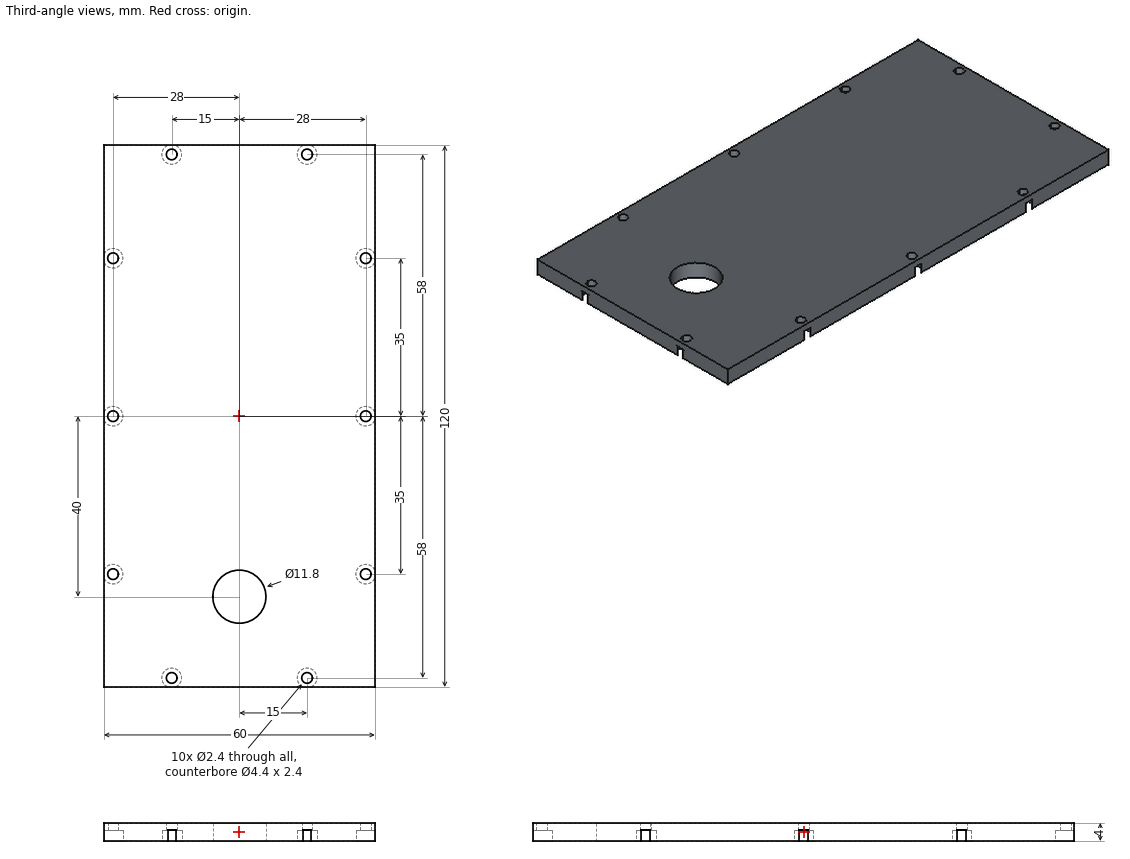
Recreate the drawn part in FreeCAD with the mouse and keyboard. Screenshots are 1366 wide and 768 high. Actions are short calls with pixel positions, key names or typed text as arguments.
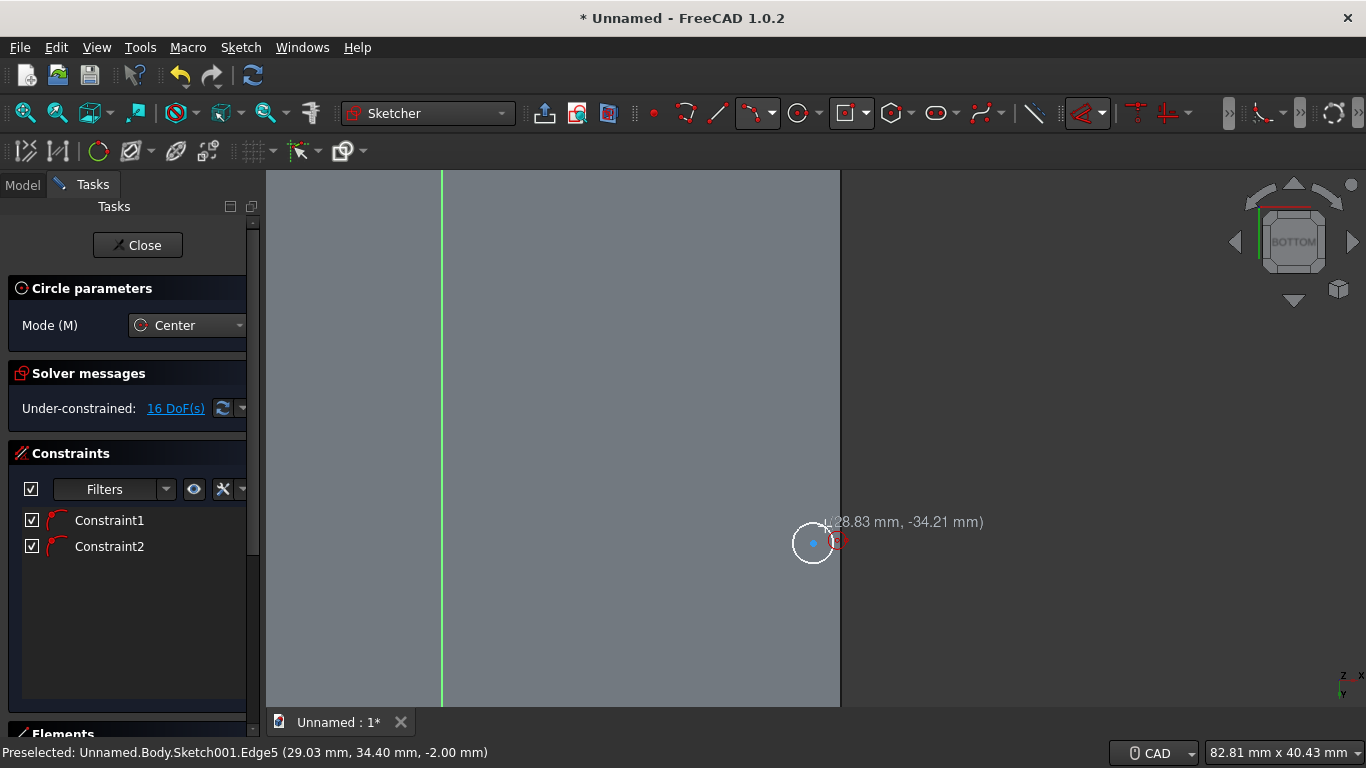
scroll(825, 531, down, 8)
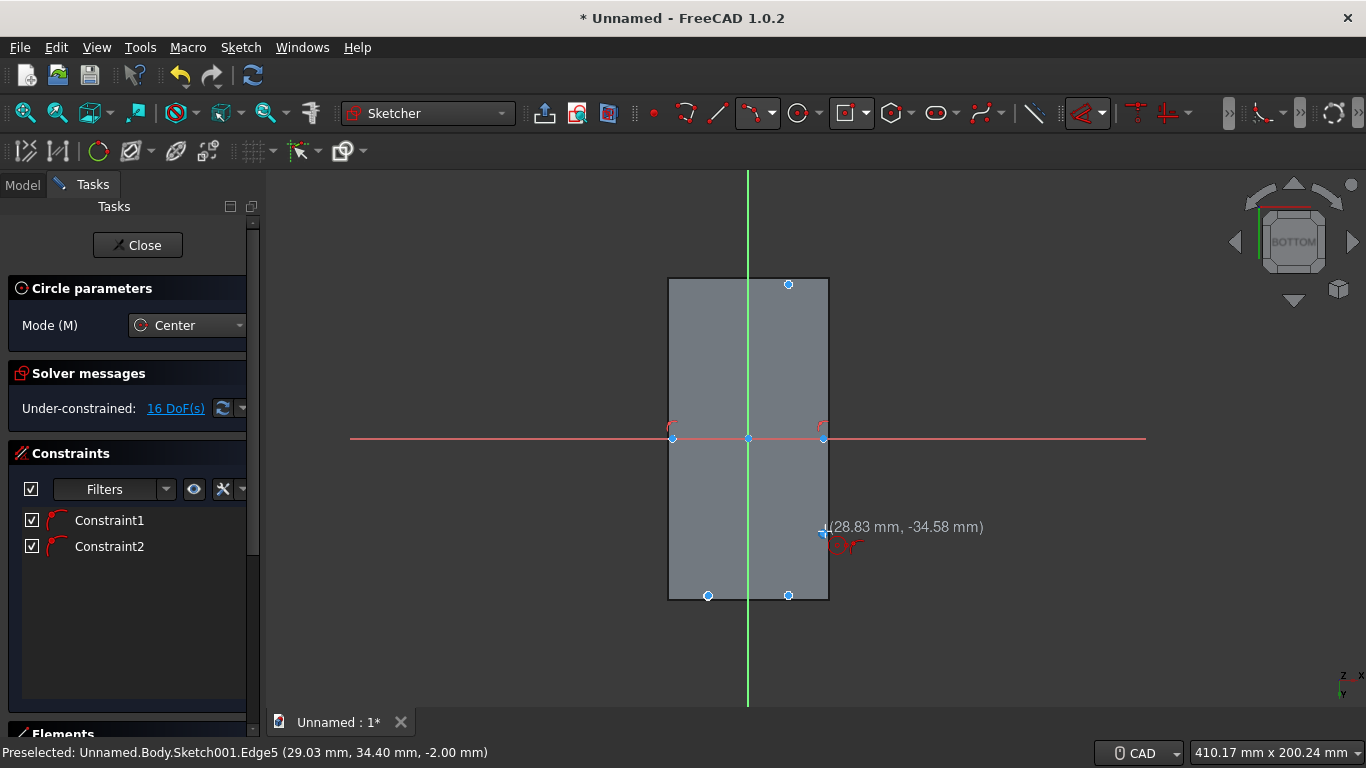
scroll(673, 533, up, 10)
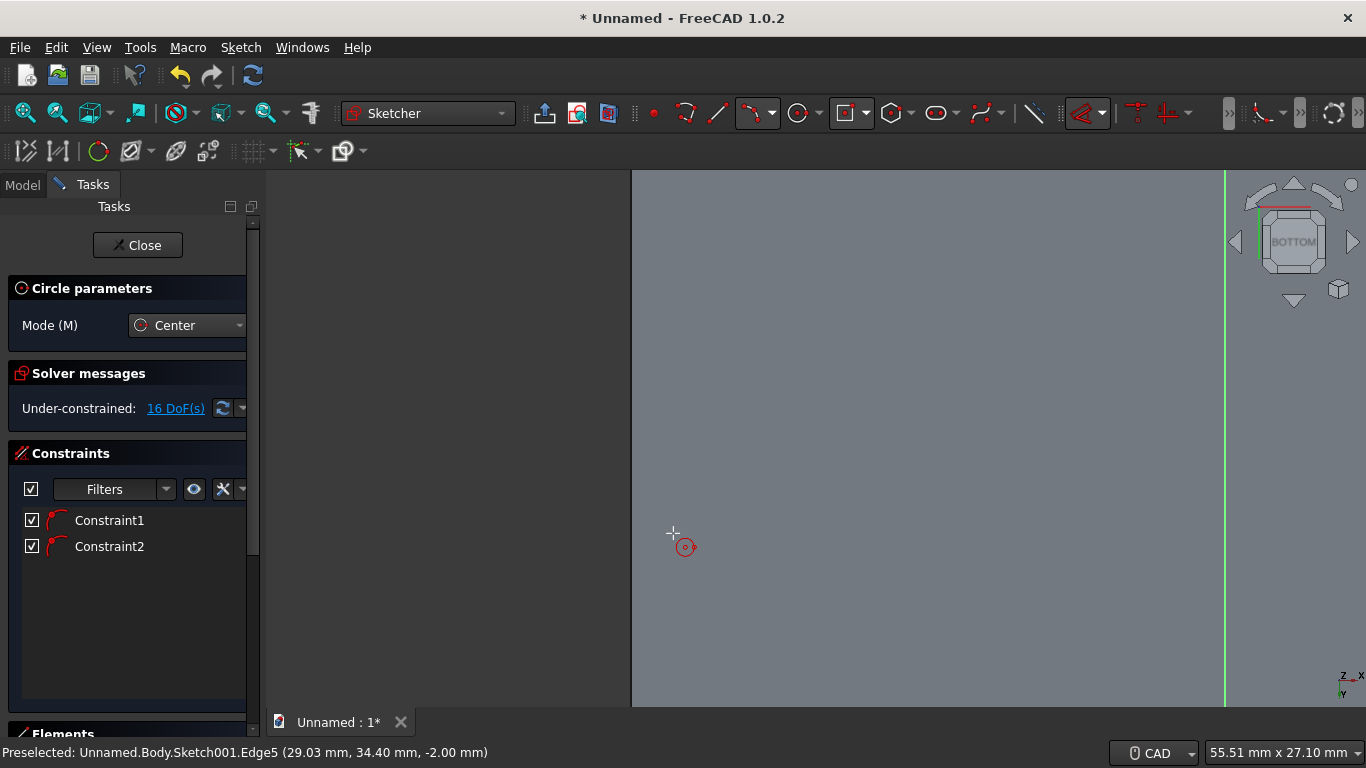
scroll(673, 533, down, 10)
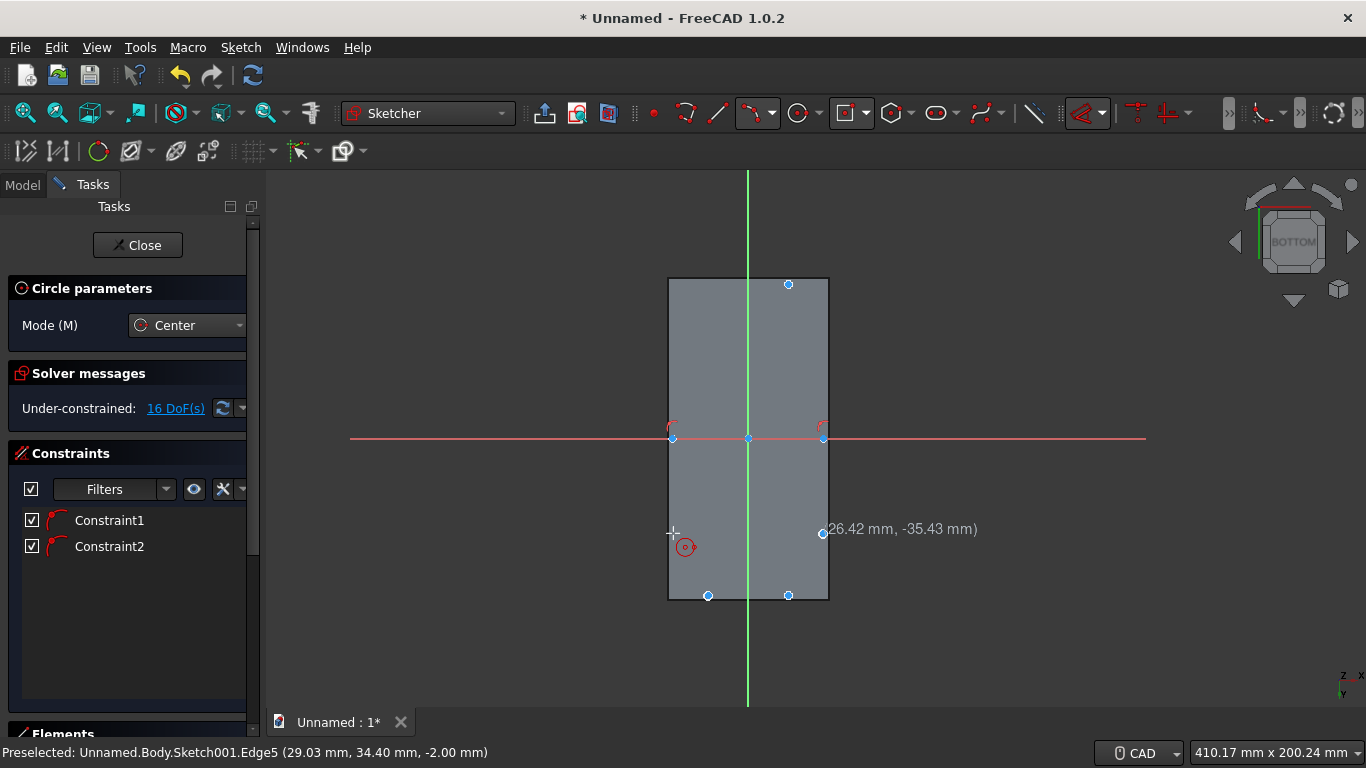
click(673, 533)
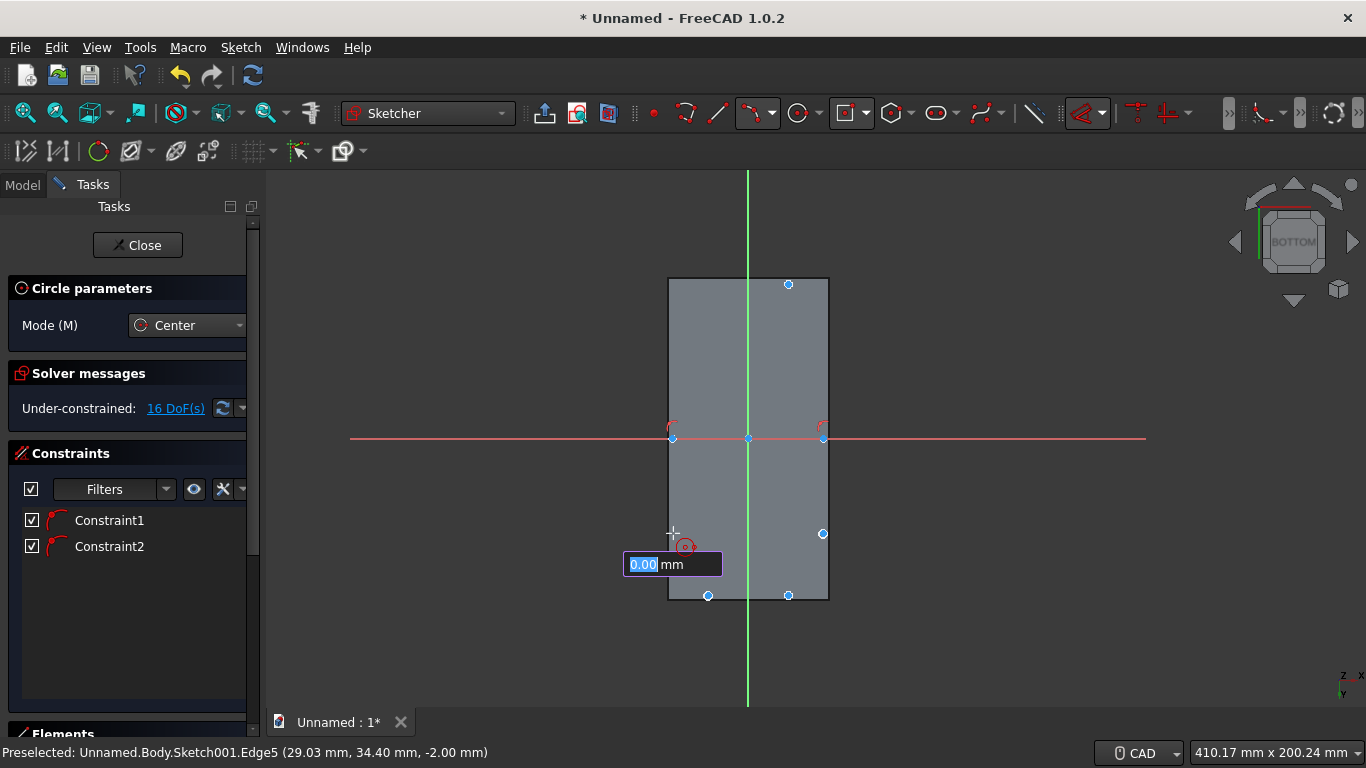
scroll(675, 531, up, 8)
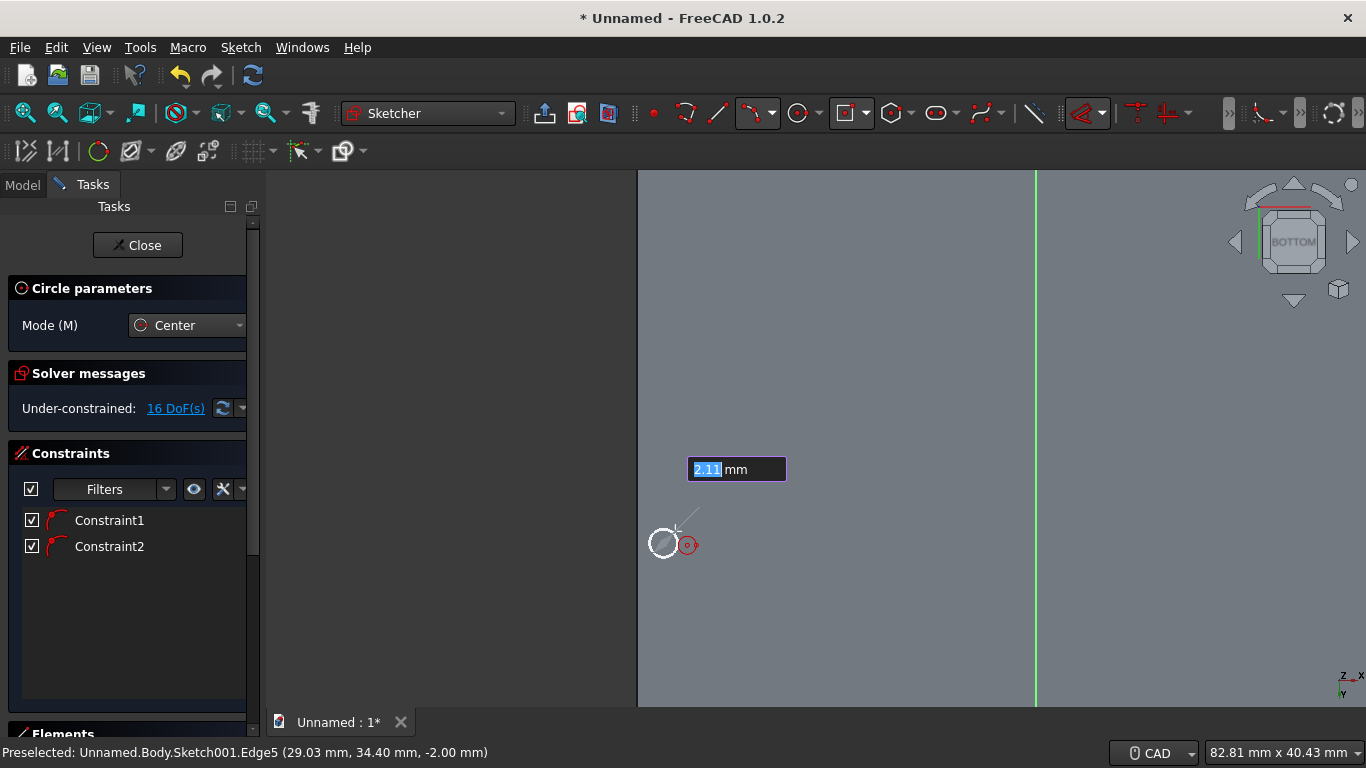
click(675, 526)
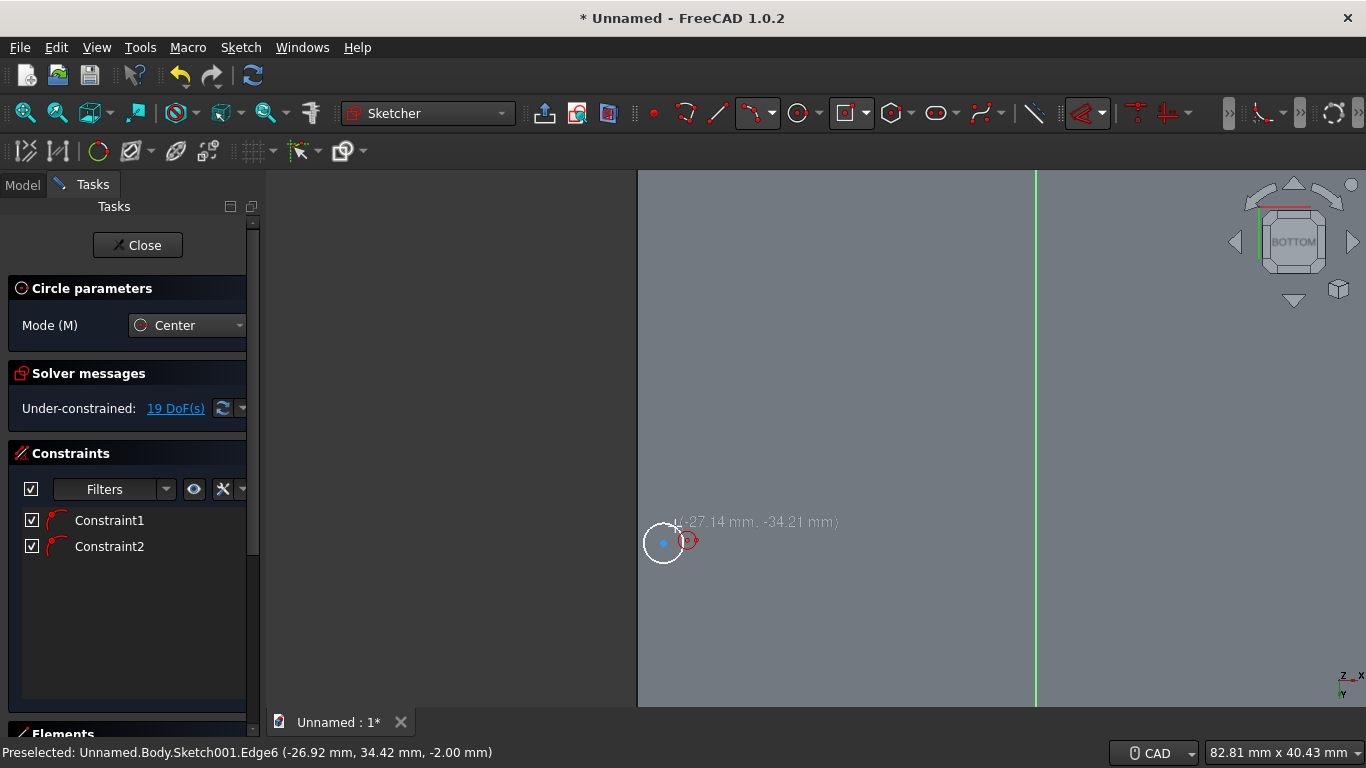
scroll(675, 531, down, 8)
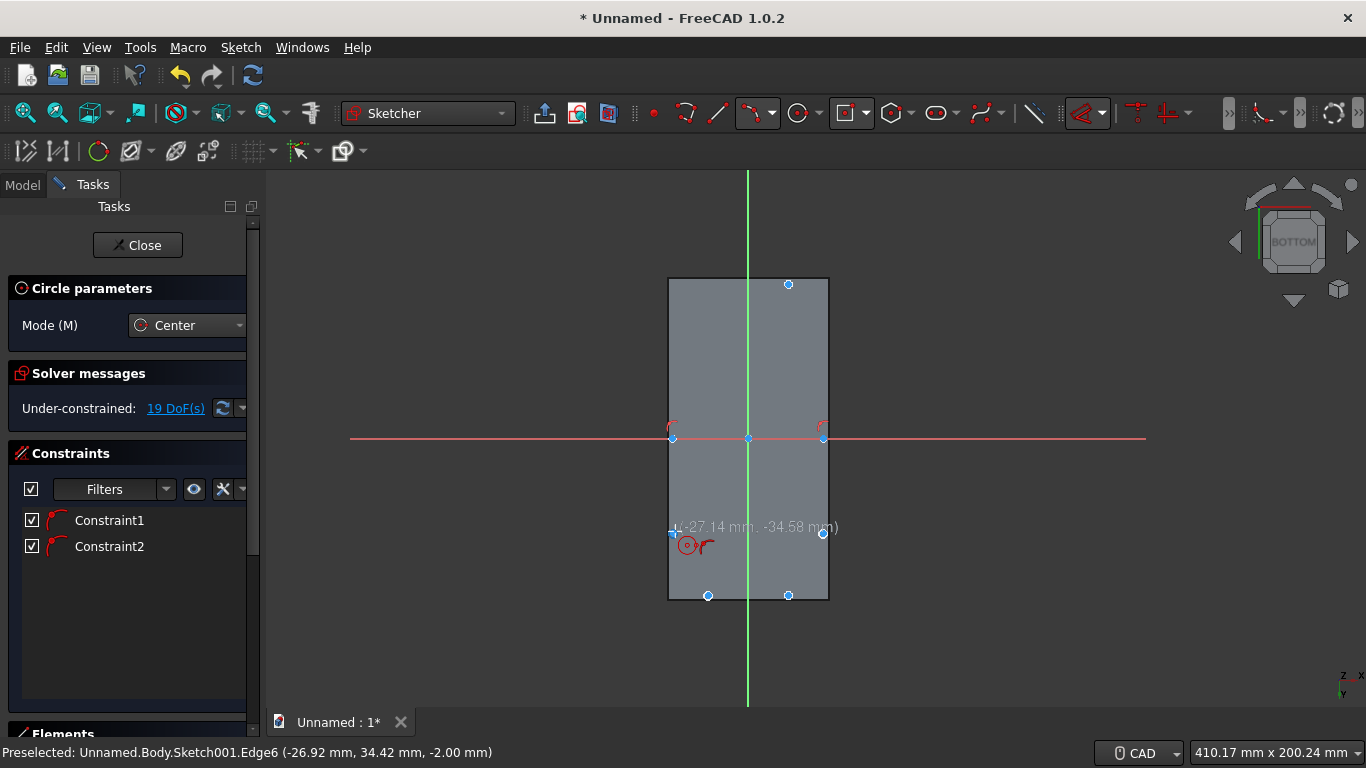
scroll(823, 345, up, 10)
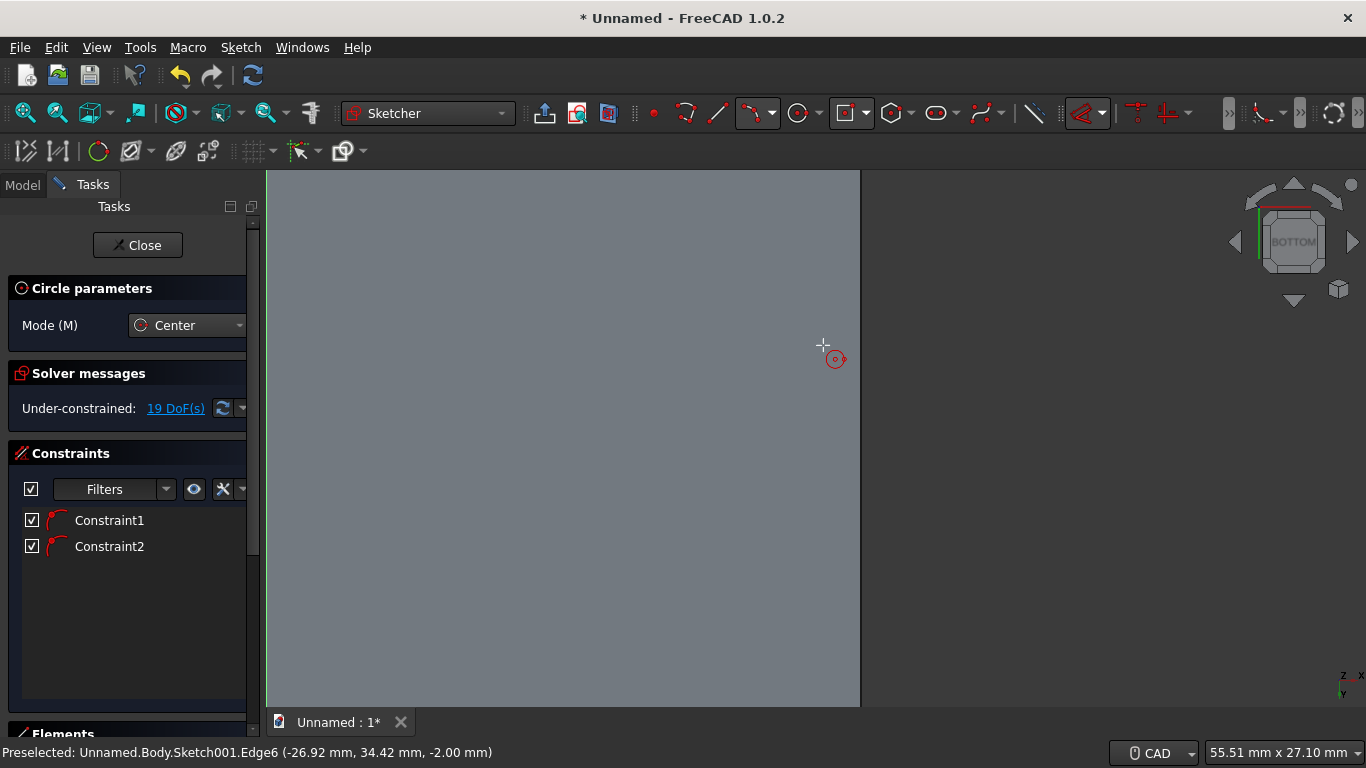
scroll(823, 345, down, 10)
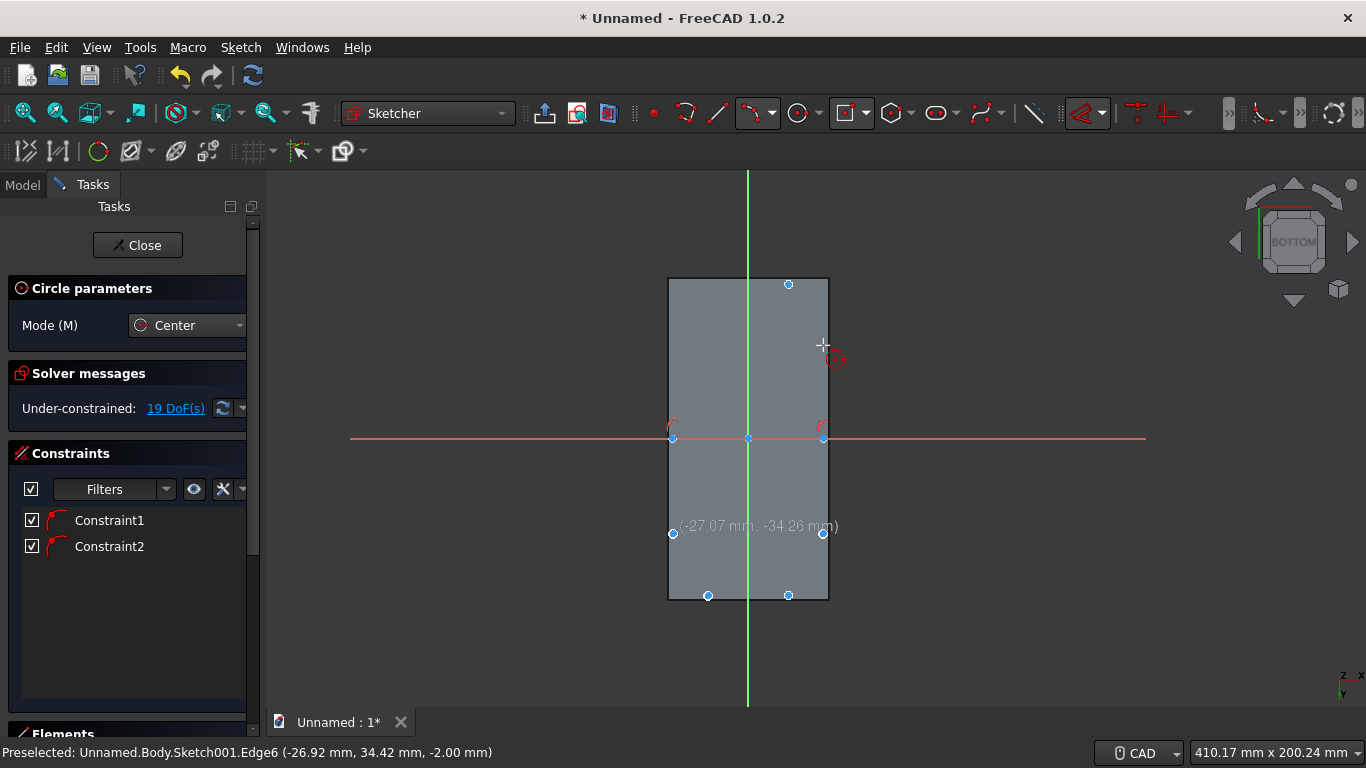
click(823, 345)